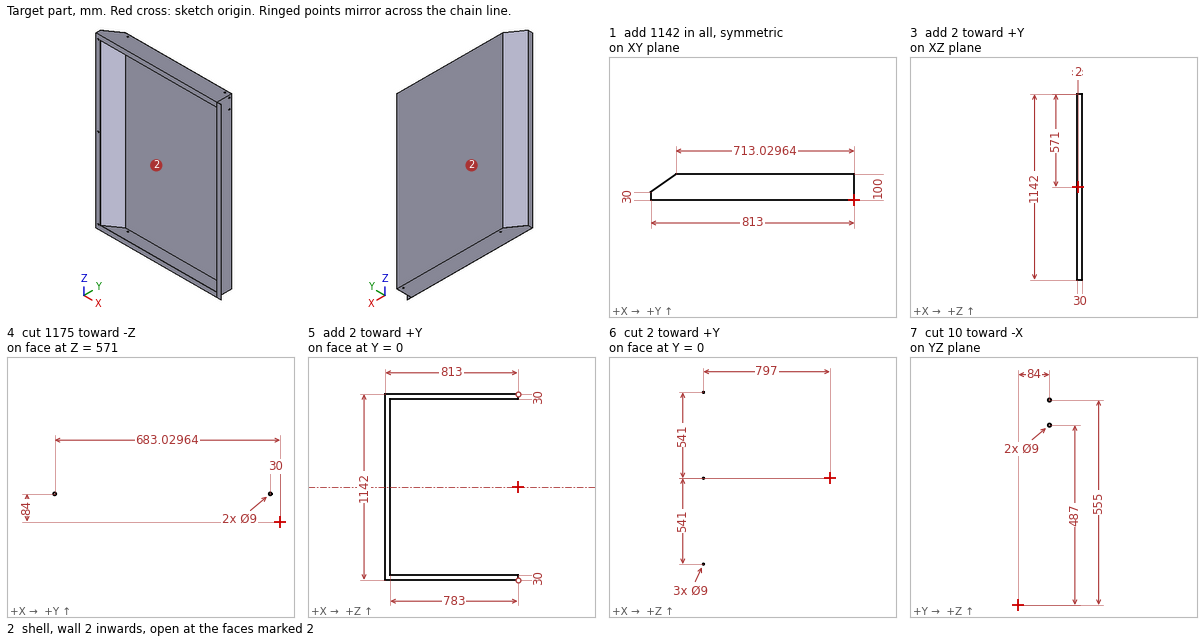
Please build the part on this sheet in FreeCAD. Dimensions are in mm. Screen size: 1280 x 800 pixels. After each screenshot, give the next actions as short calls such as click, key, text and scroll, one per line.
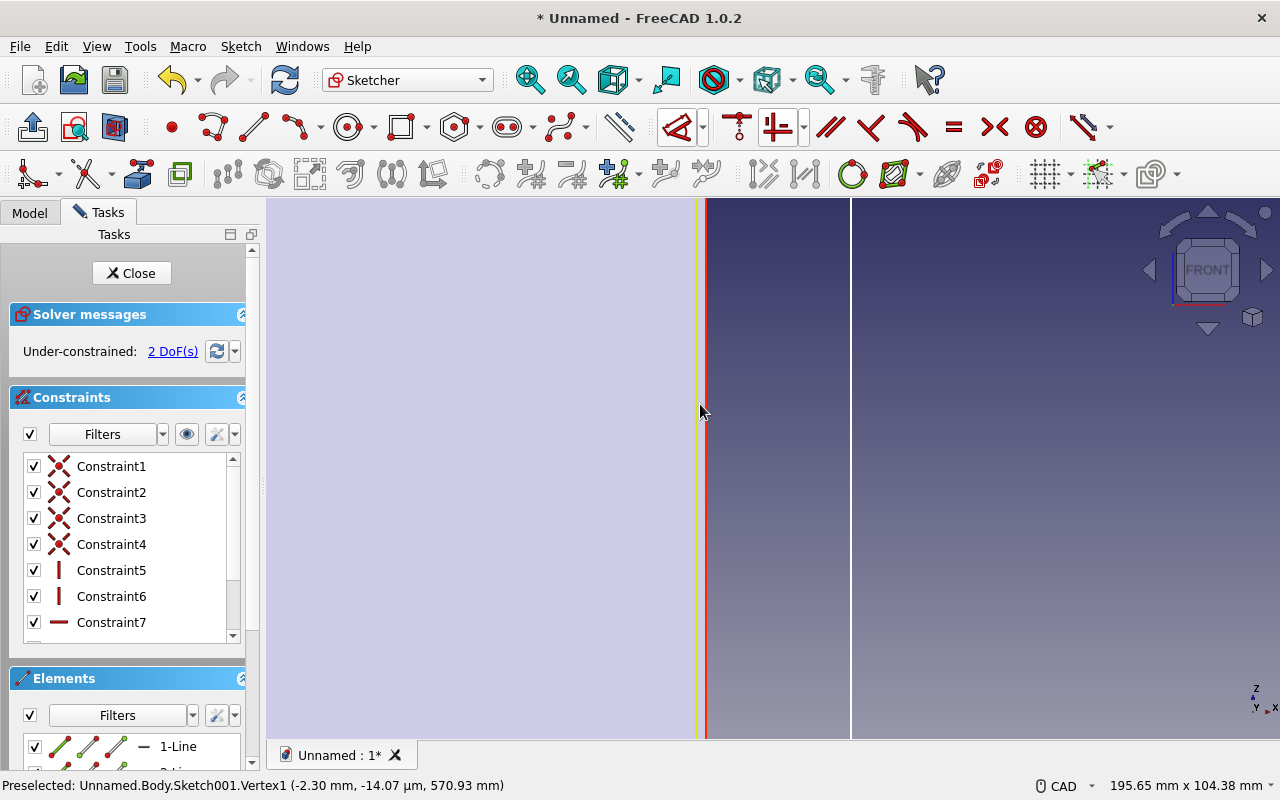
click(696, 404)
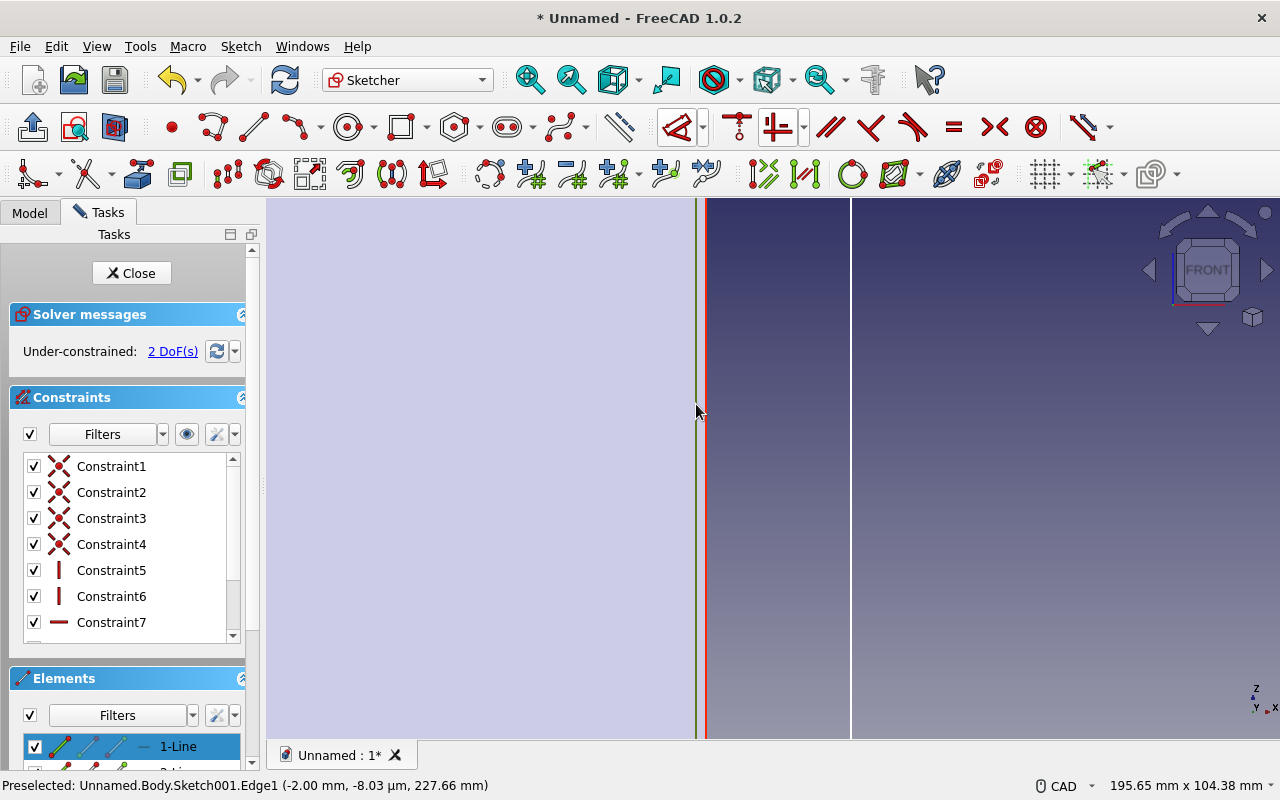
click(702, 128)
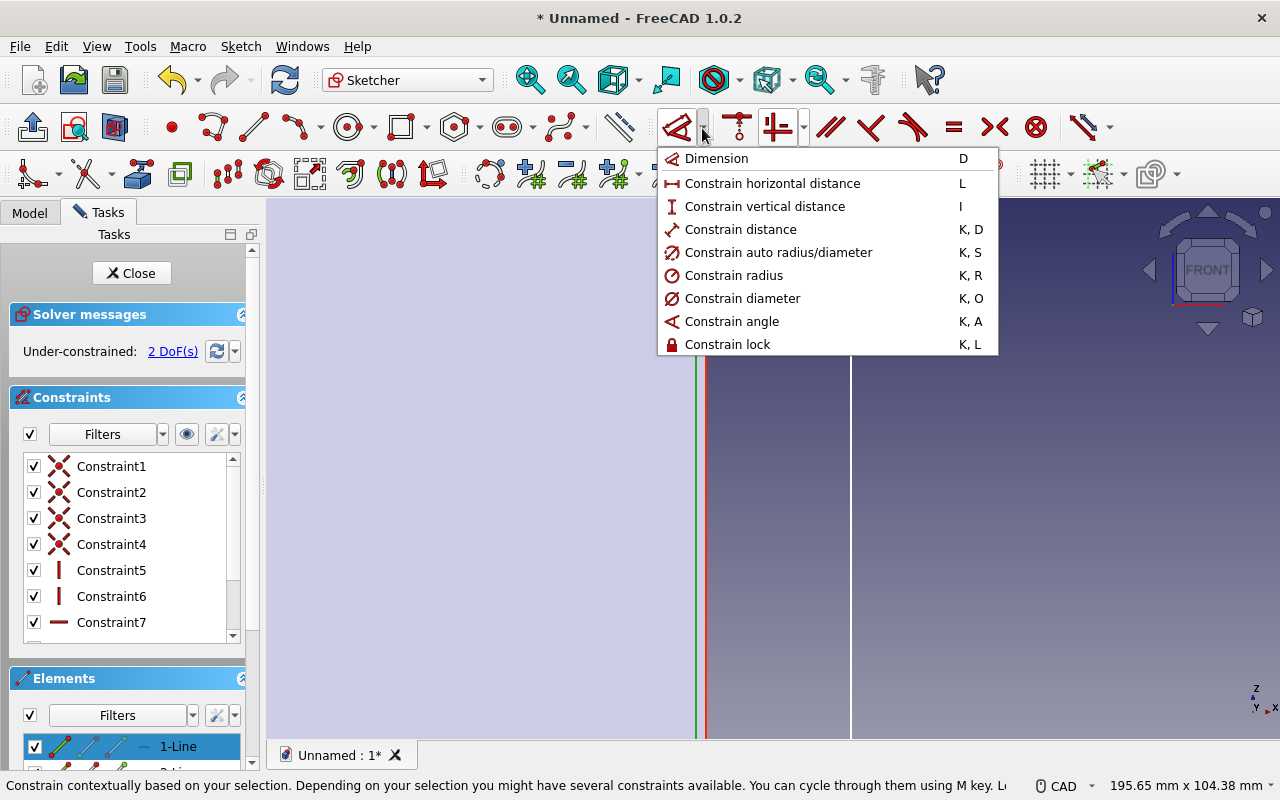
click(828, 206)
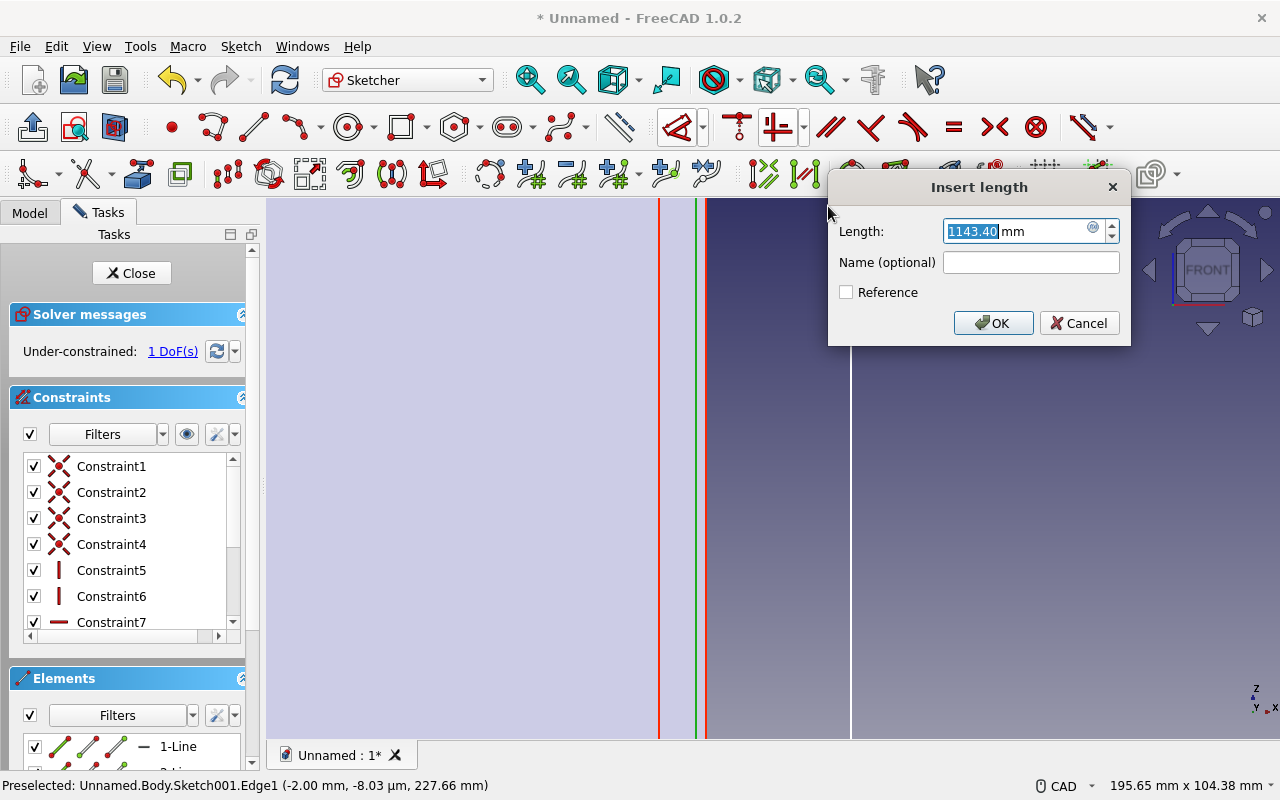
text(1142)
key(Return)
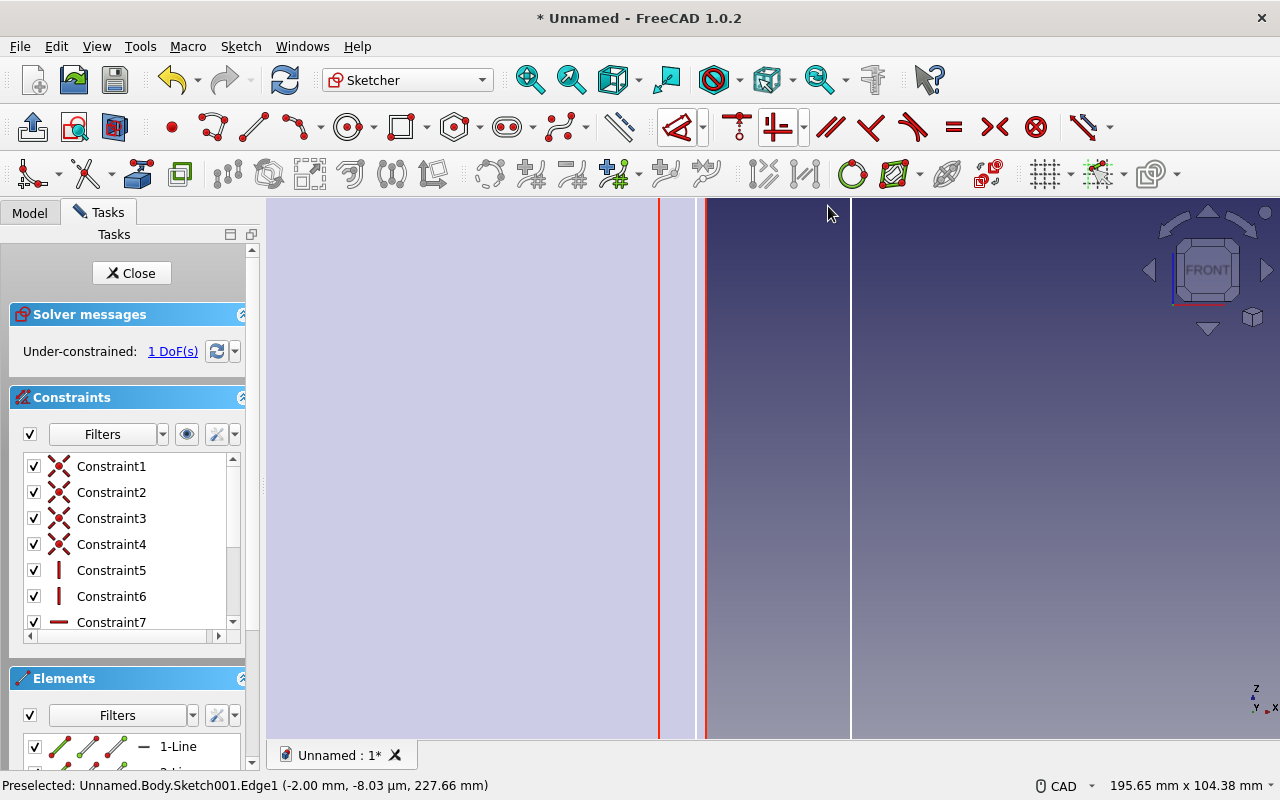
scroll(700, 396, down, 14)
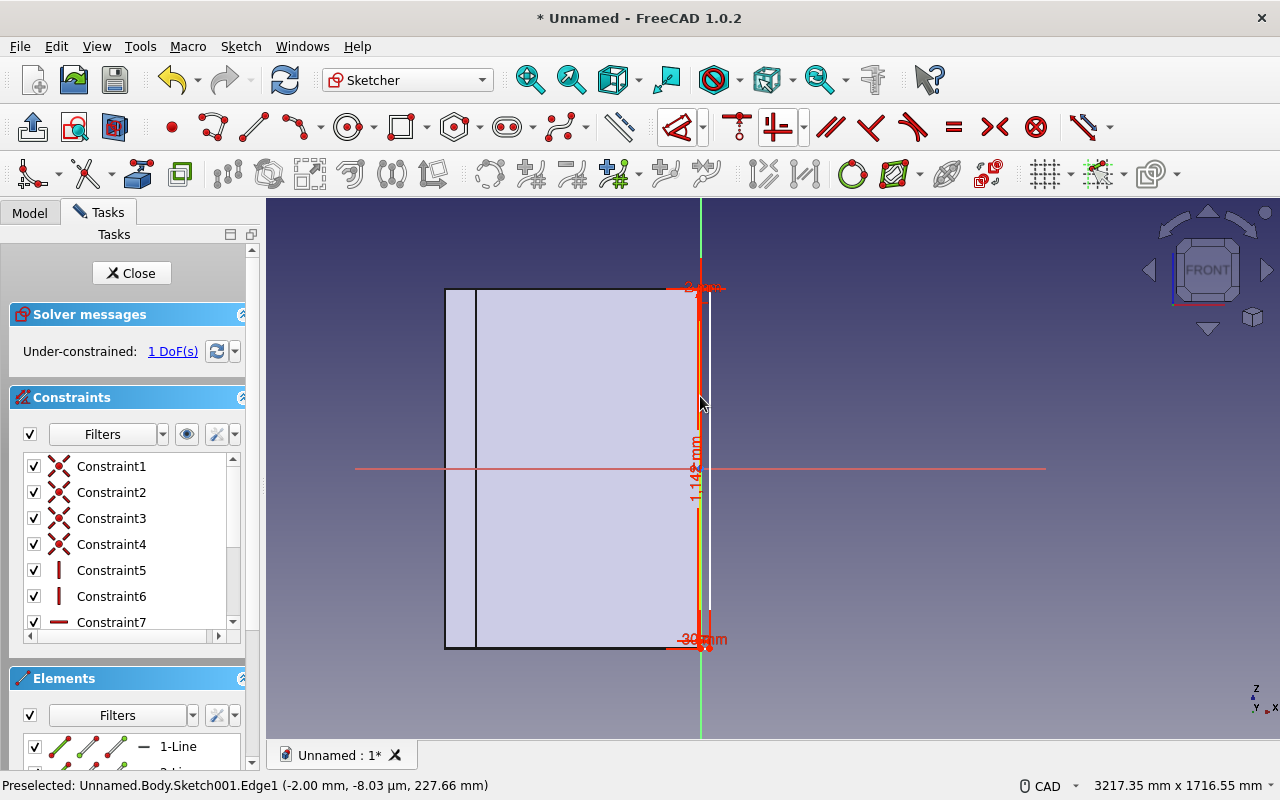
scroll(700, 289, up, 2)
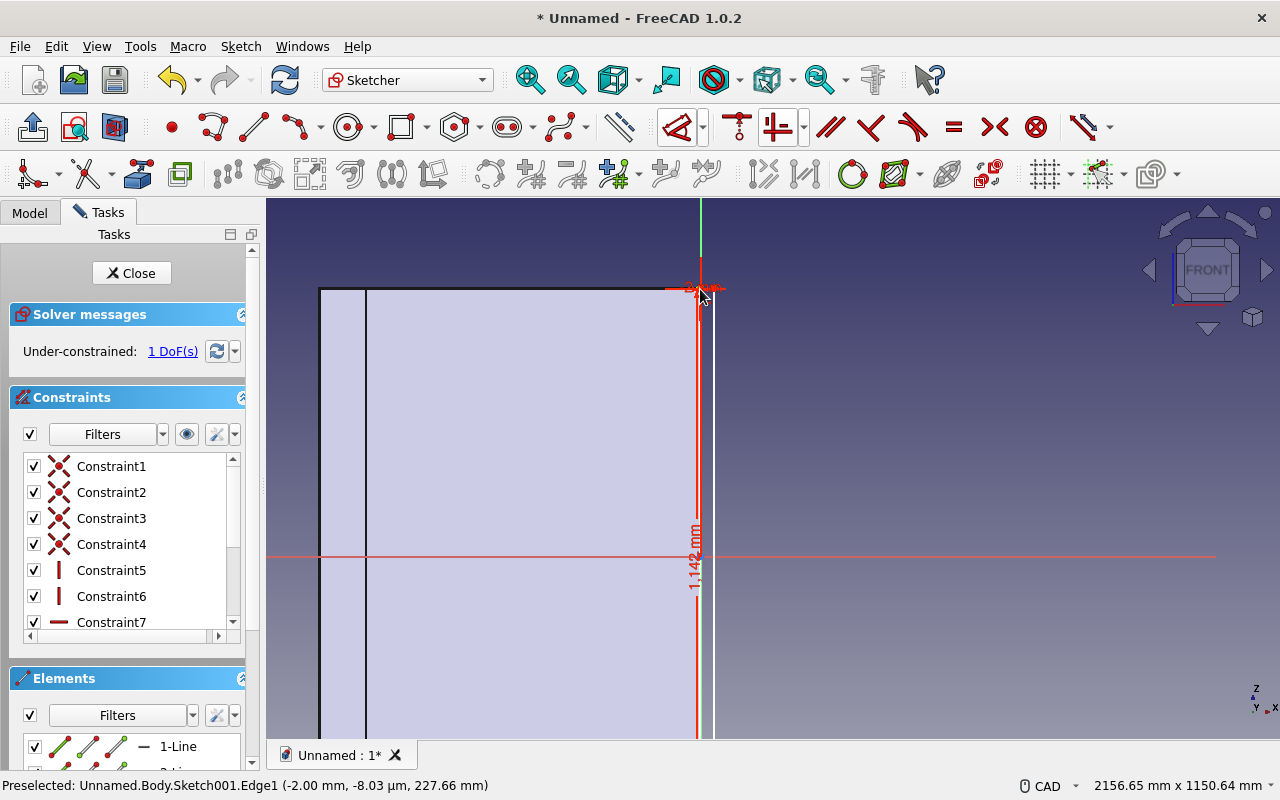
click(700, 289)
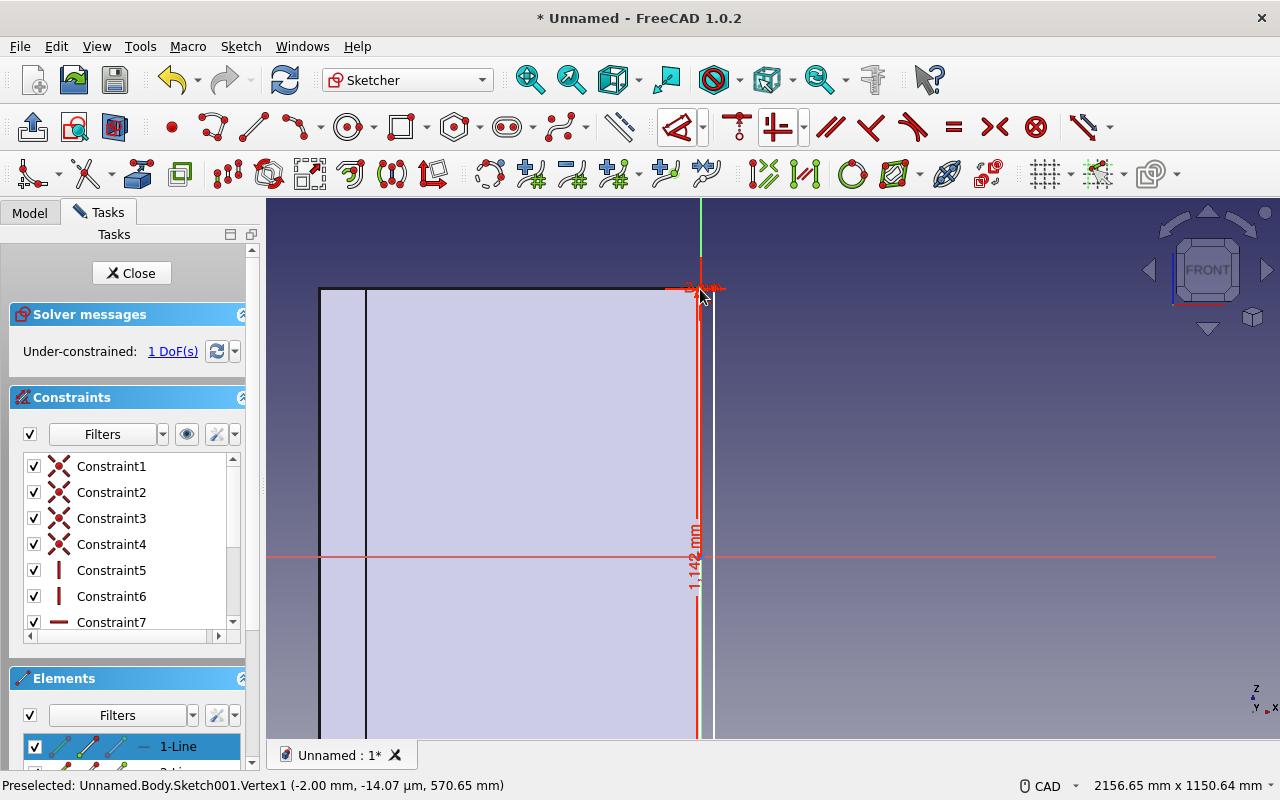
click(702, 128)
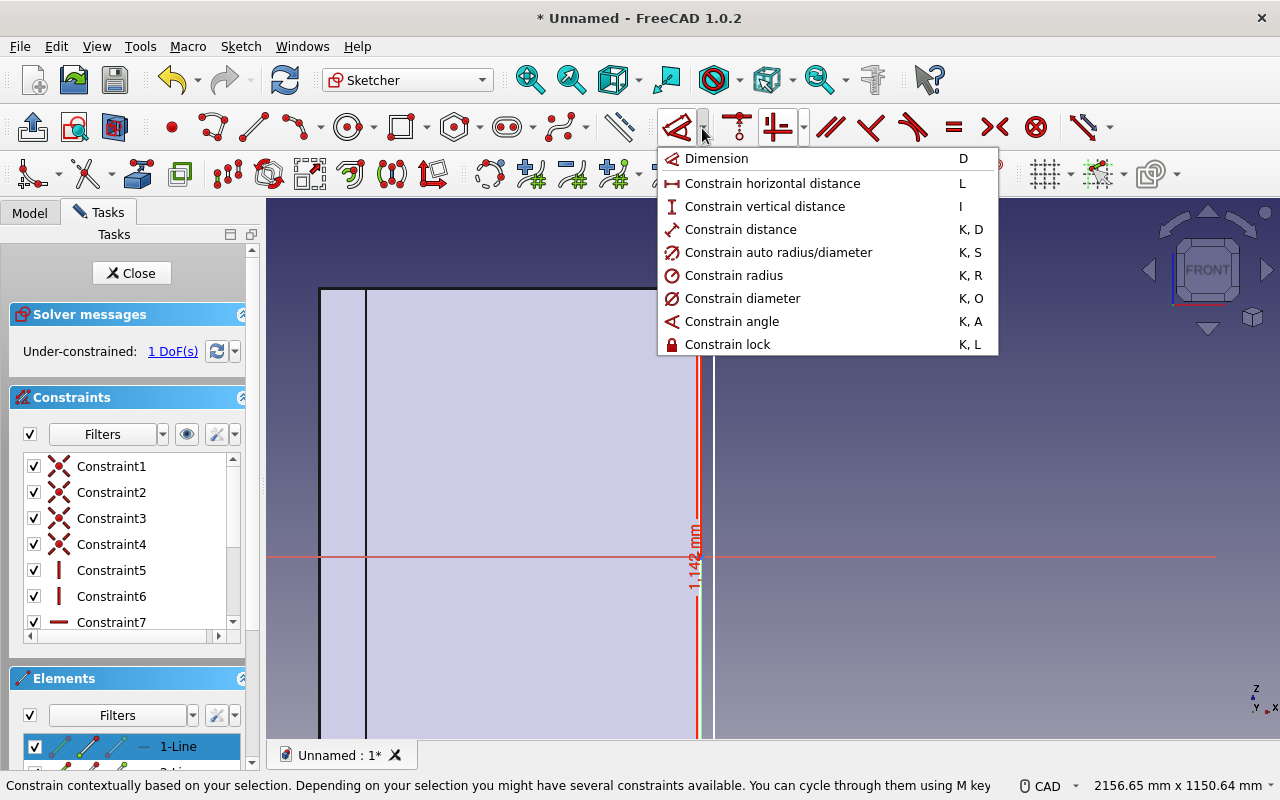
click(828, 206)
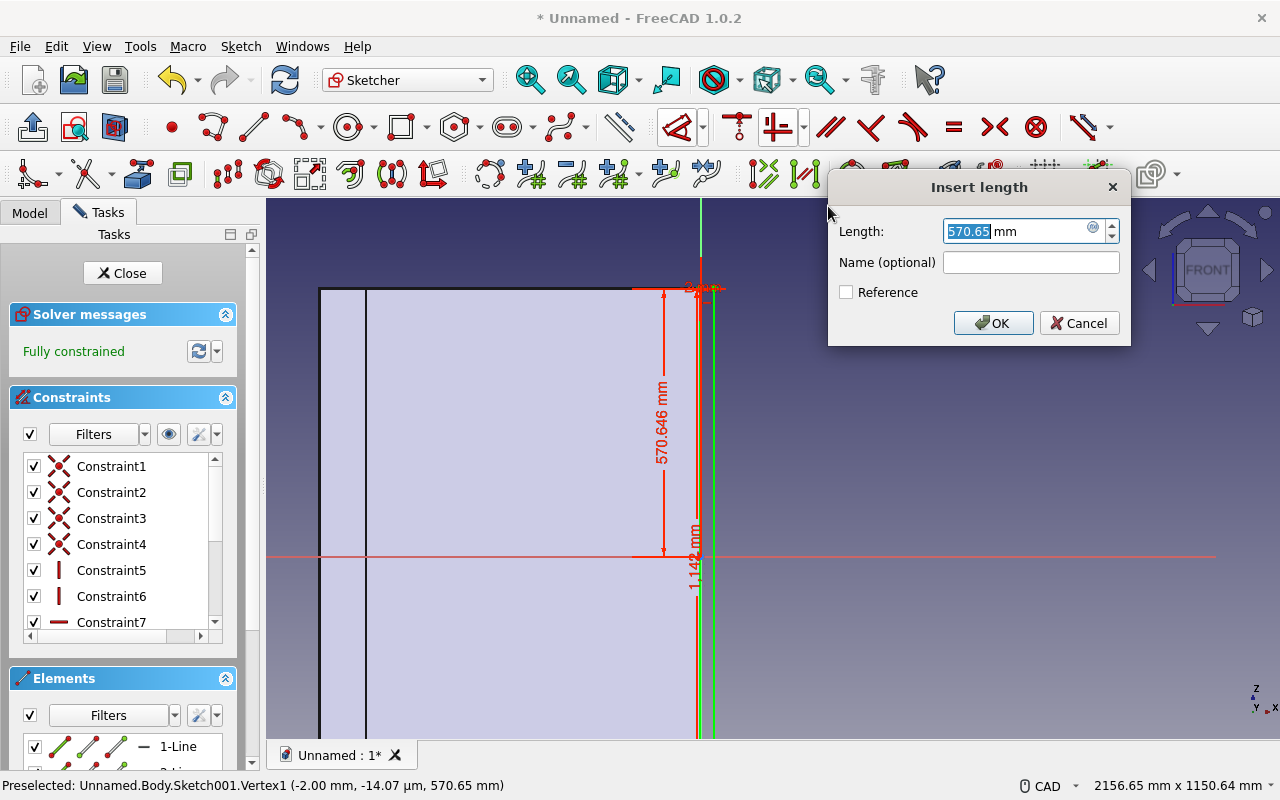
text(571)
key(Return)